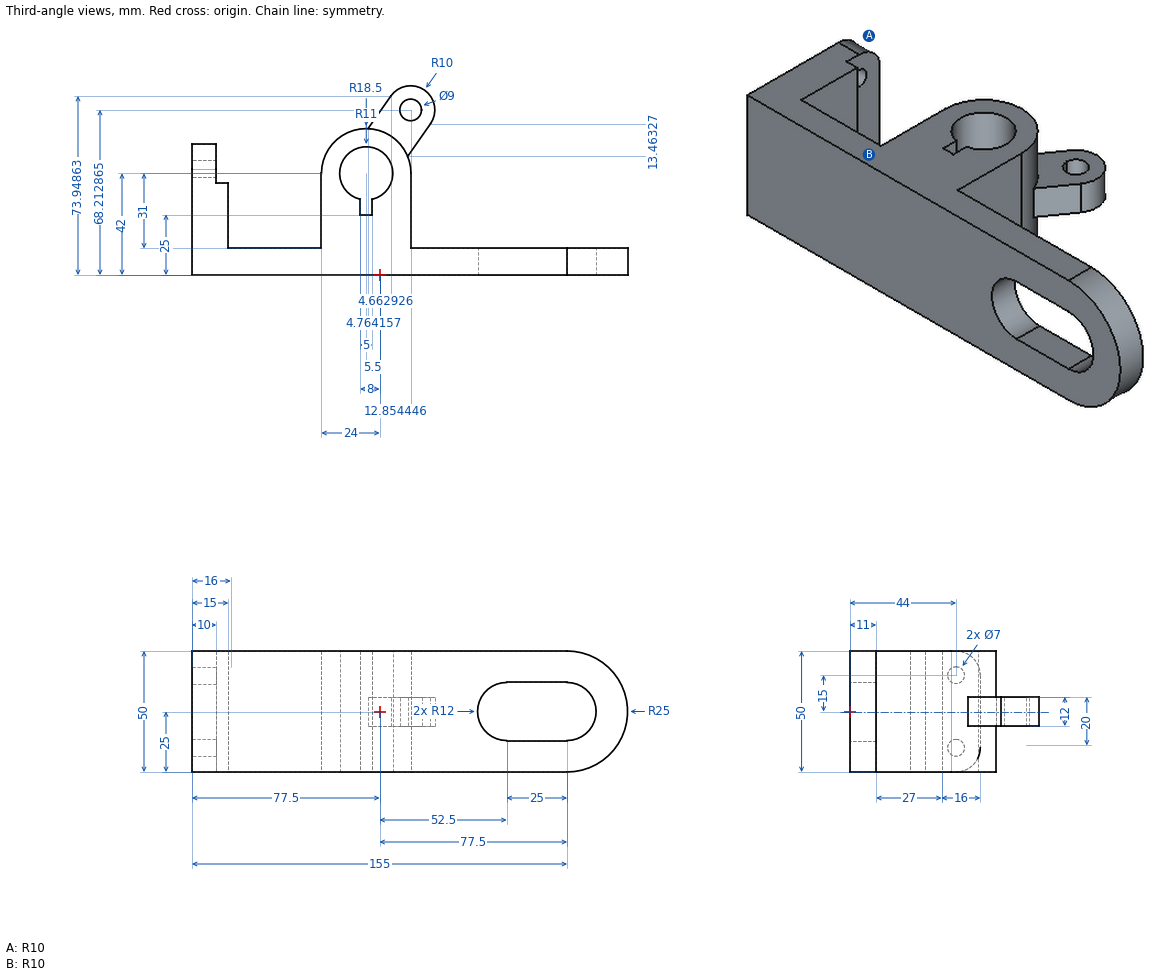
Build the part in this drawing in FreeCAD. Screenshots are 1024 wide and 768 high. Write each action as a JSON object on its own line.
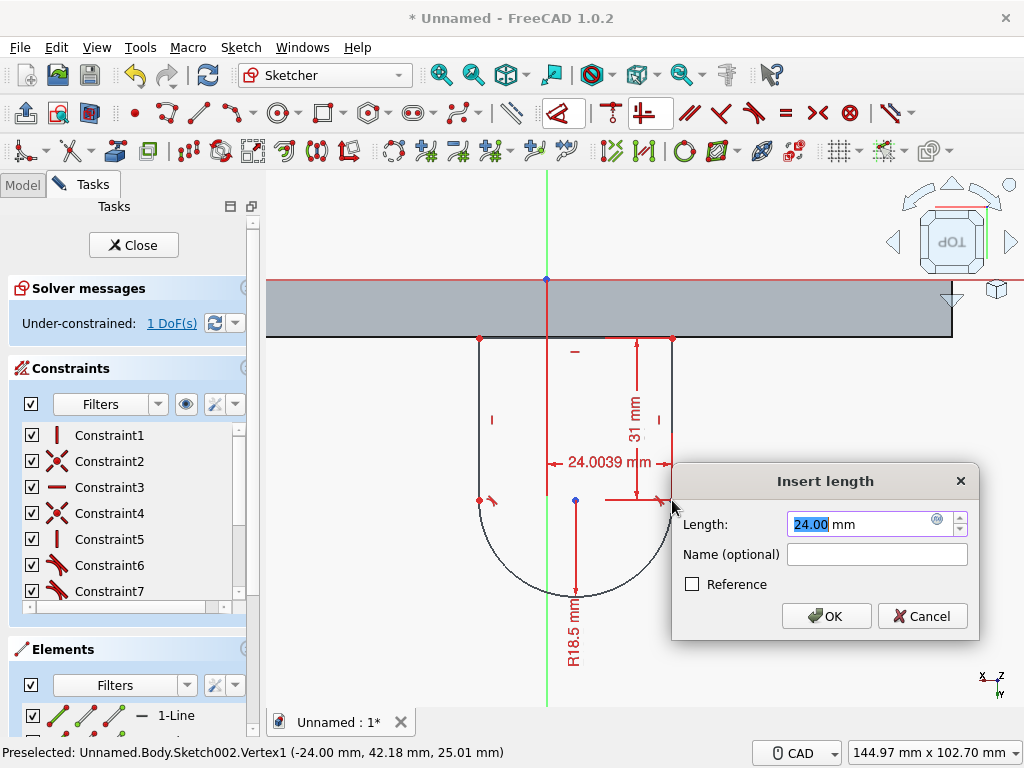
{"action": "type", "text": "24"}
{"action": "key", "text": "Return"}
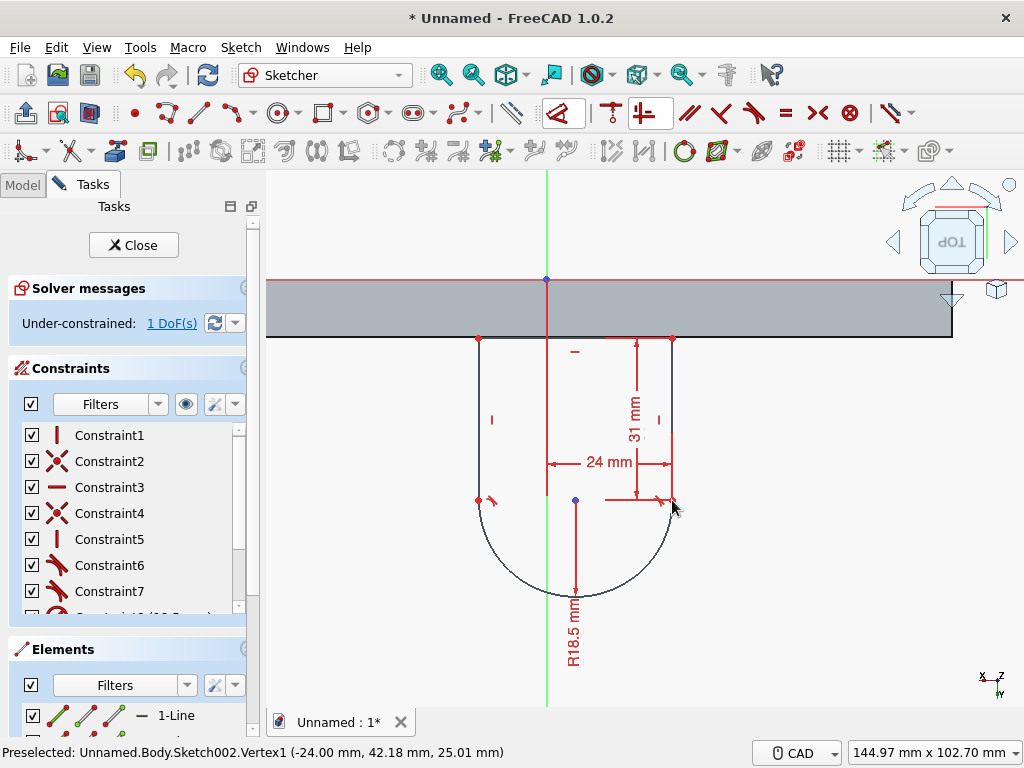
{"action": "left_click", "coordinate": [672, 500]}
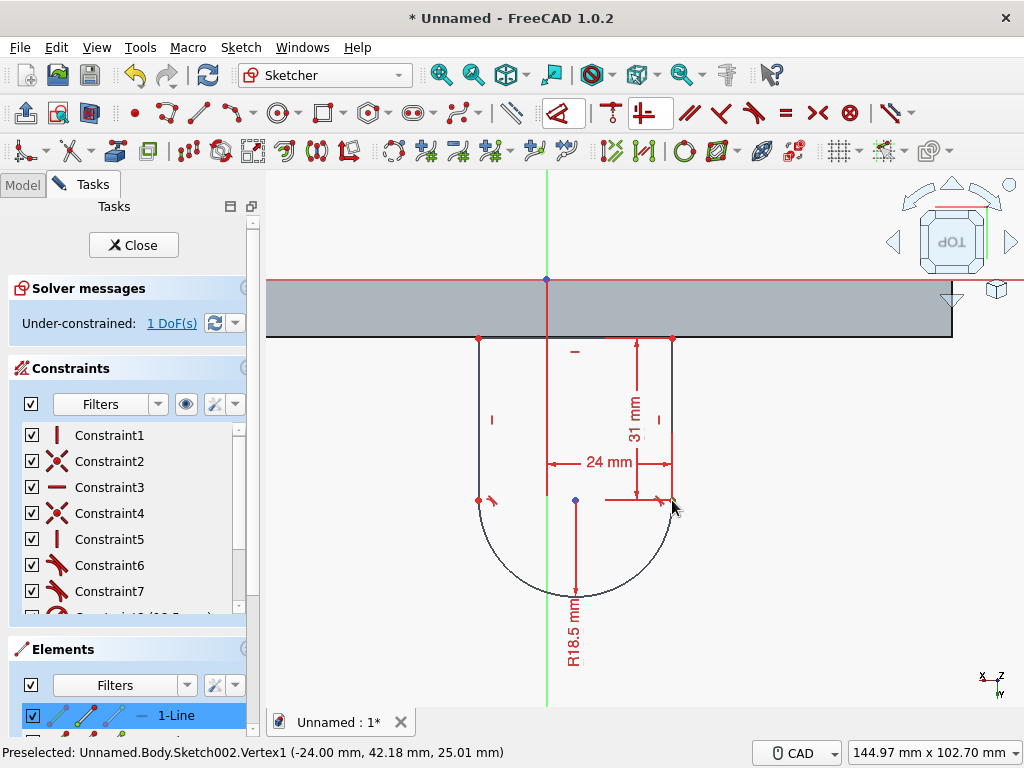
{"action": "left_click", "coordinate": [580, 114]}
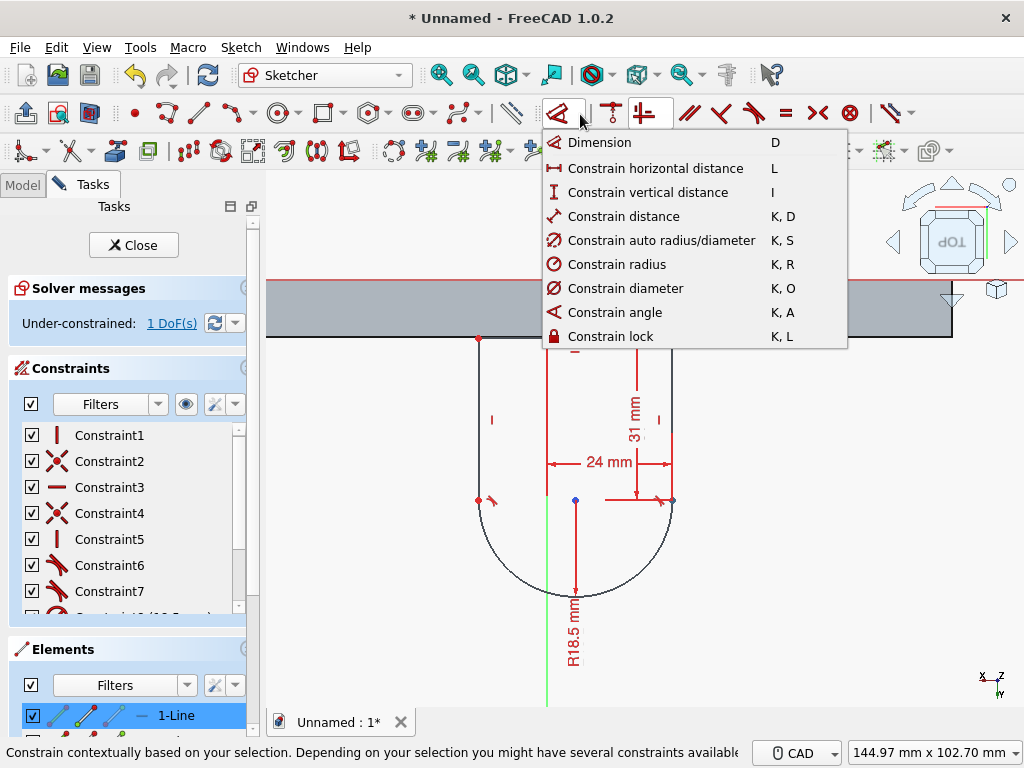
{"action": "left_click", "coordinate": [695, 192]}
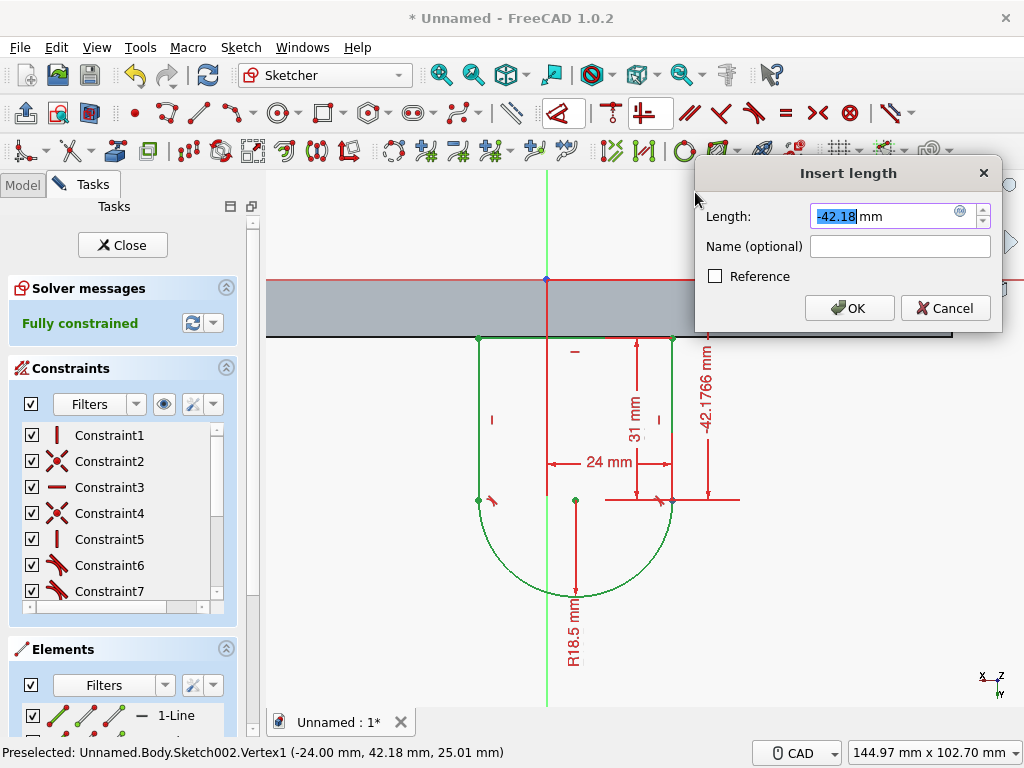
{"action": "type", "text": "-42"}
{"action": "key", "text": "Return"}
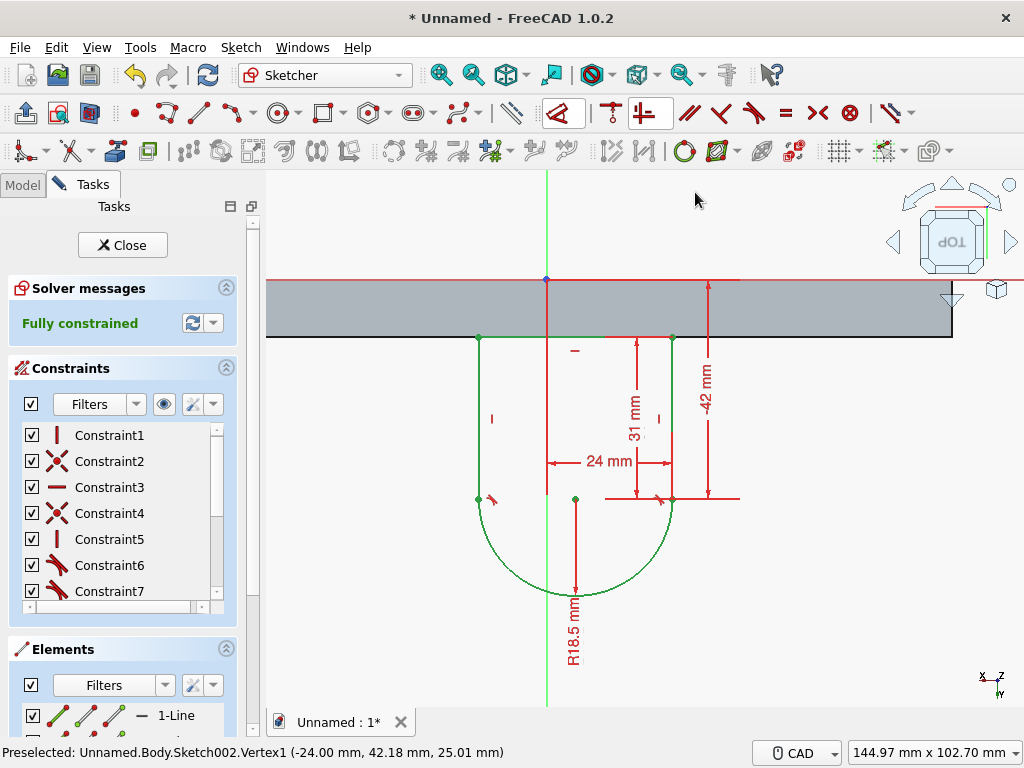
{"action": "left_click", "coordinate": [123, 245]}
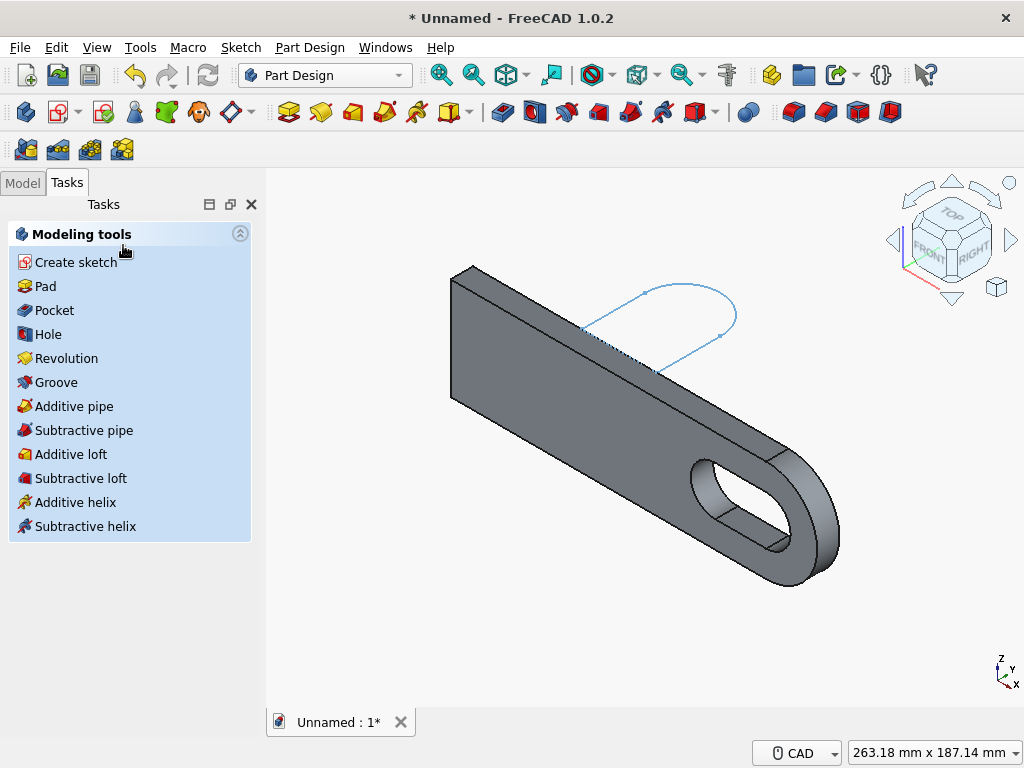
{"action": "left_click", "coordinate": [290, 112]}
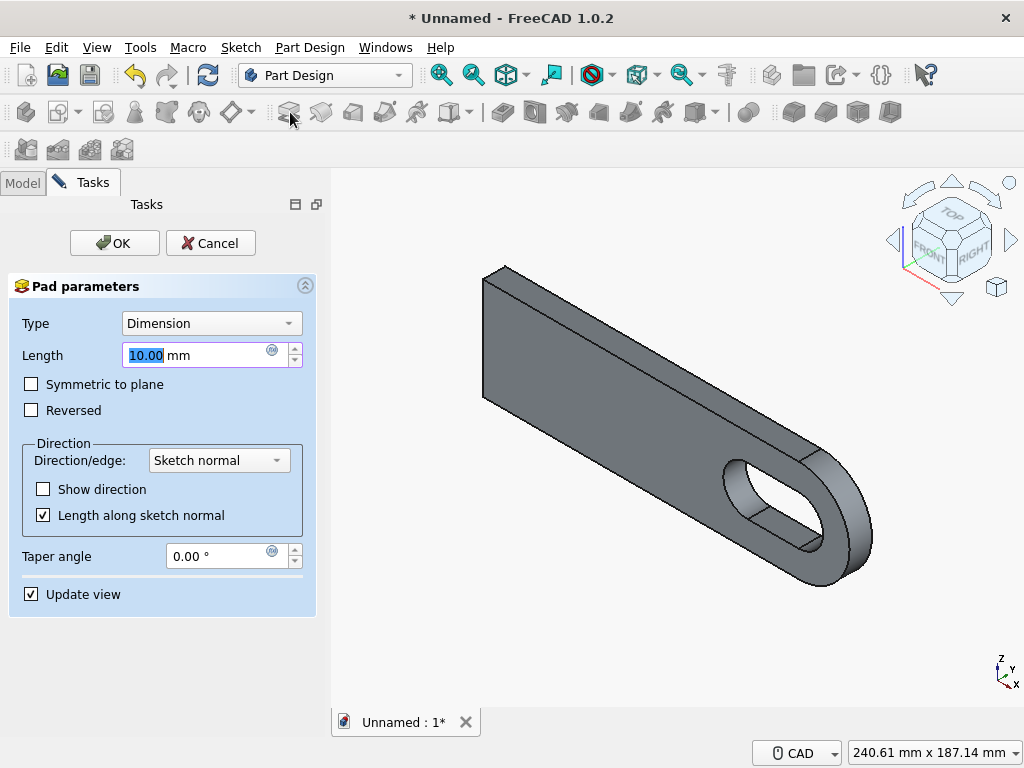
{"action": "type", "text": "50"}
{"action": "key", "text": "Tab"}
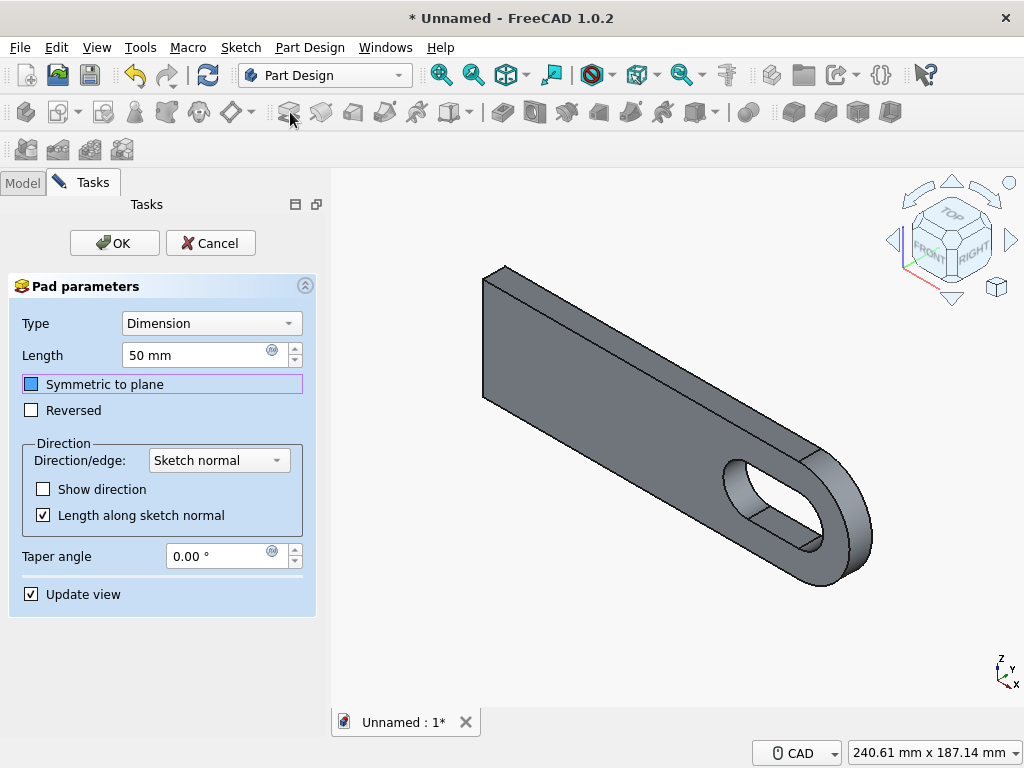
{"action": "left_click", "coordinate": [30, 410]}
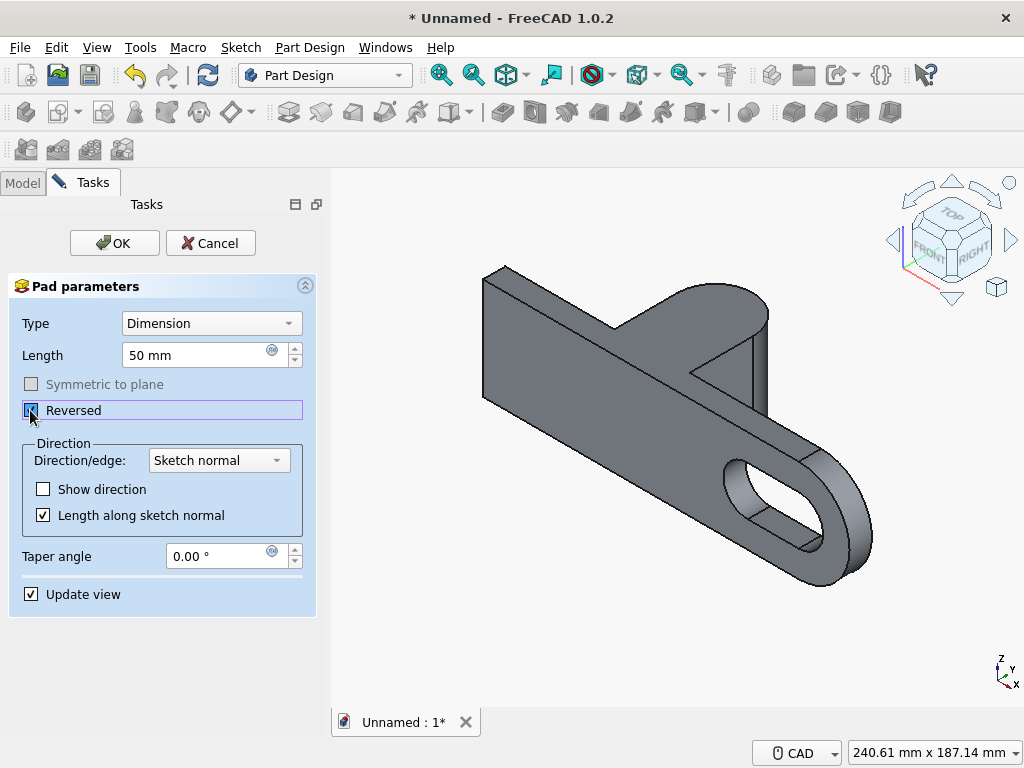
{"action": "left_click", "coordinate": [115, 243]}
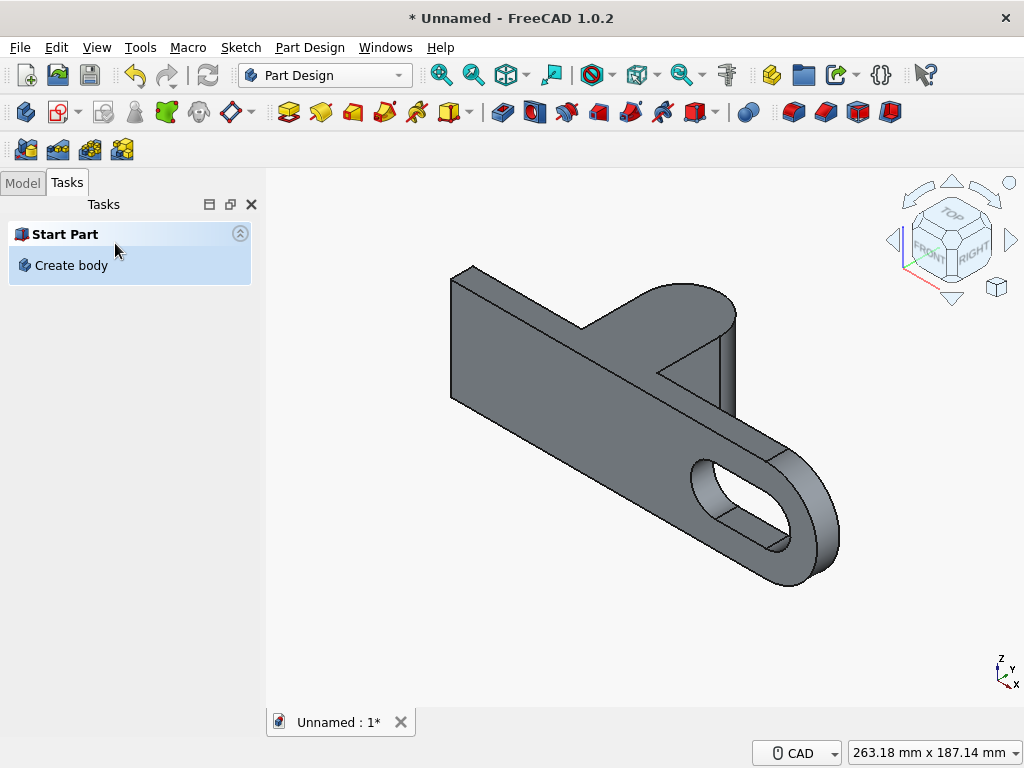
{"action": "left_click", "coordinate": [688, 324]}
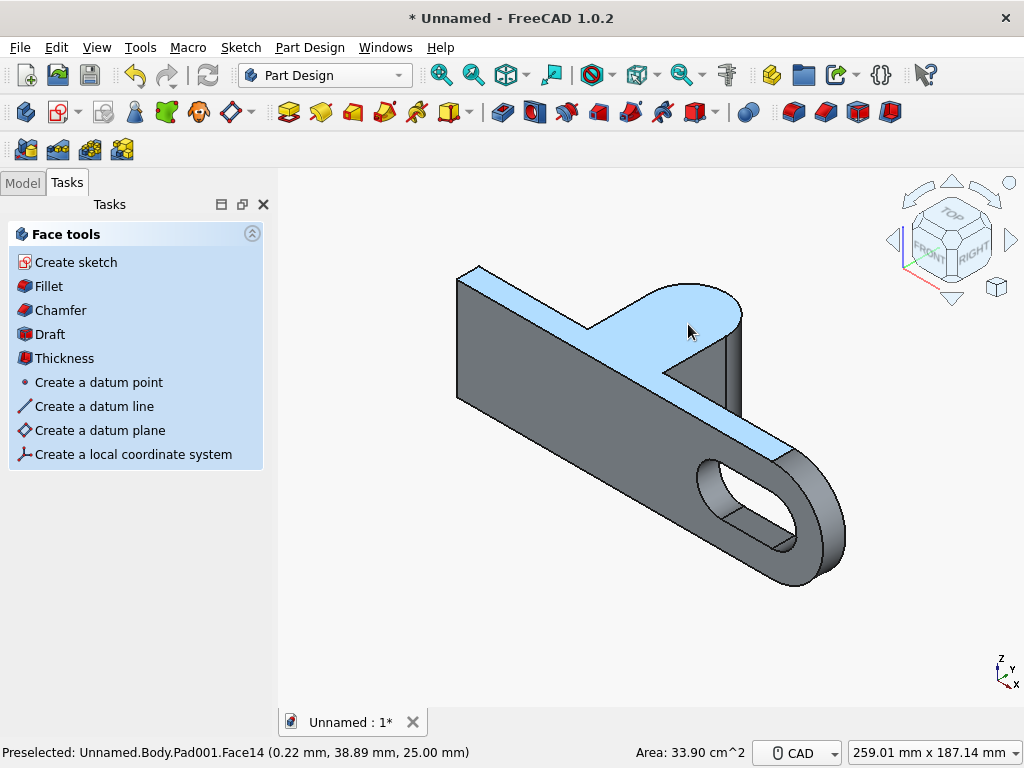
{"action": "left_click", "coordinate": [58, 112]}